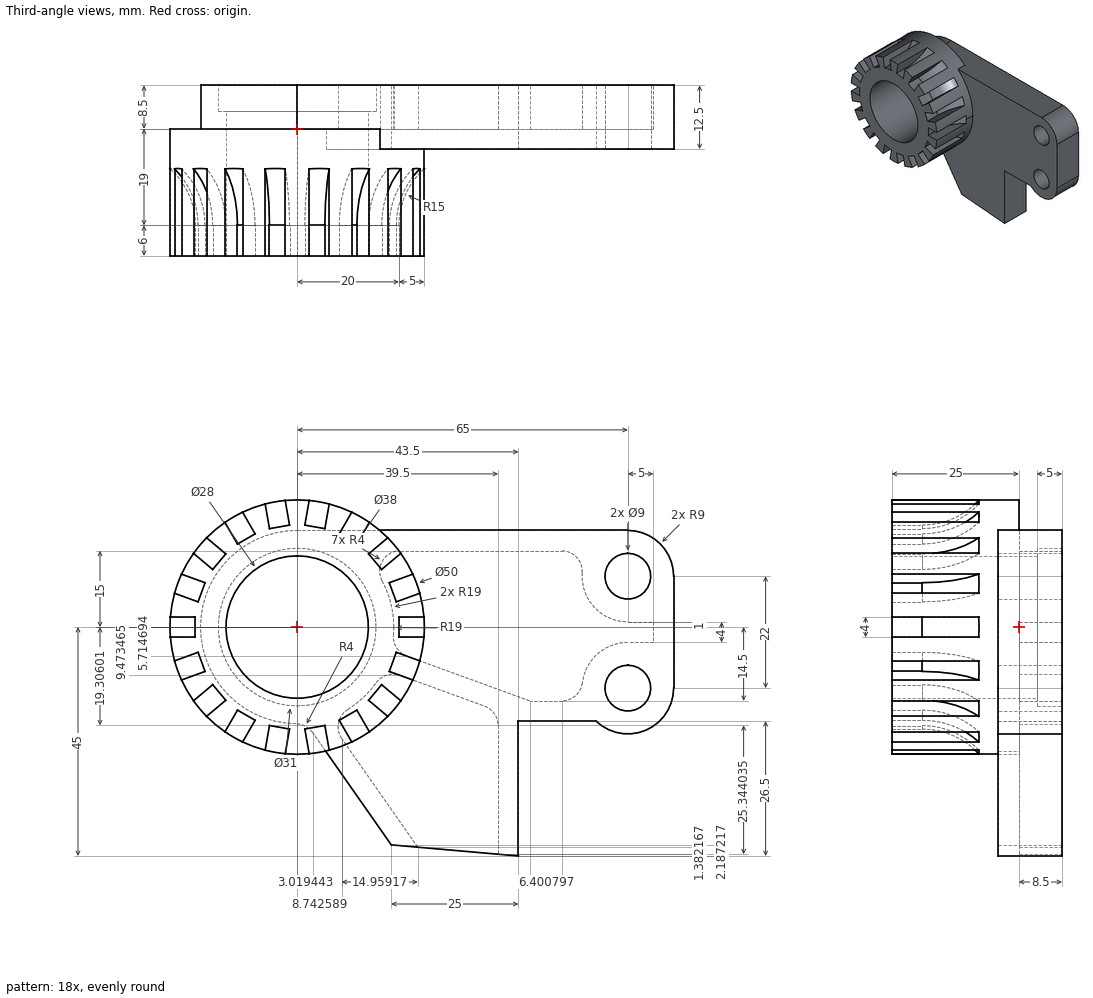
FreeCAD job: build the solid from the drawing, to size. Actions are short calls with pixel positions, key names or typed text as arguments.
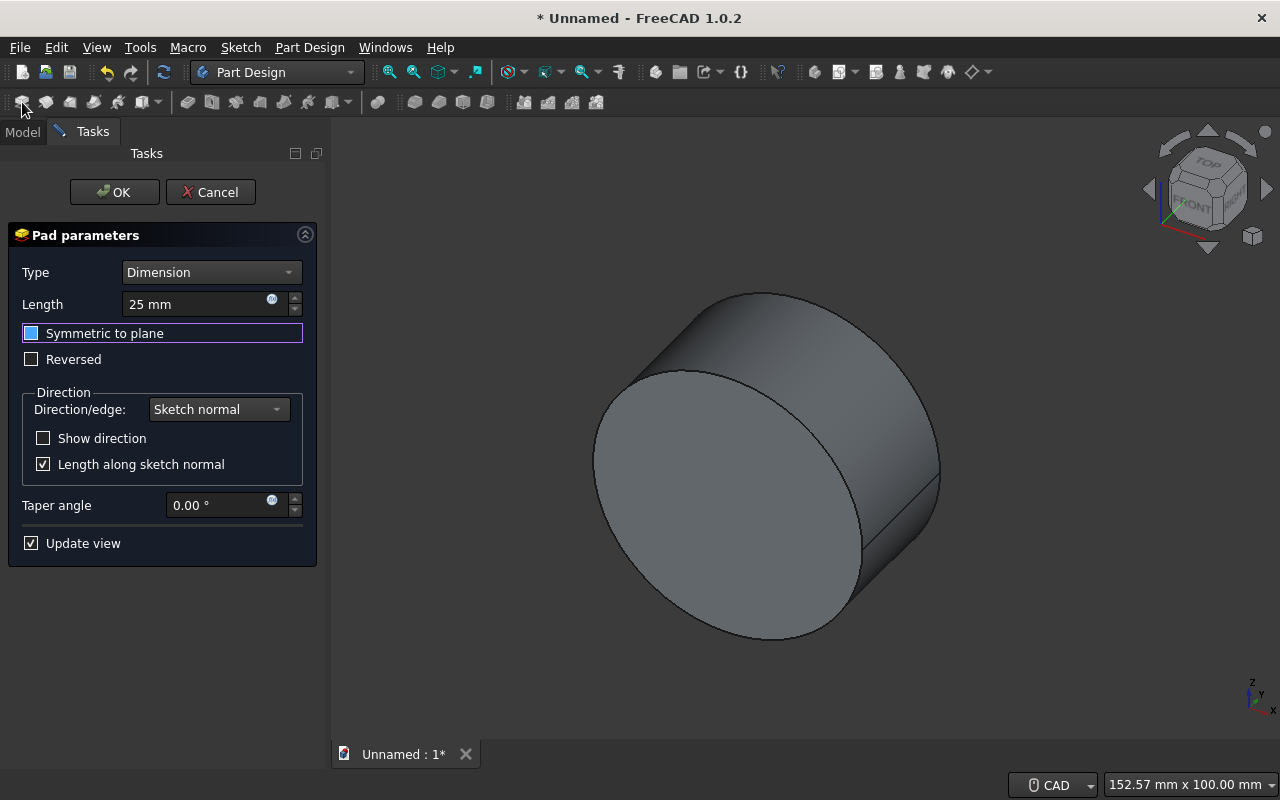
click(115, 192)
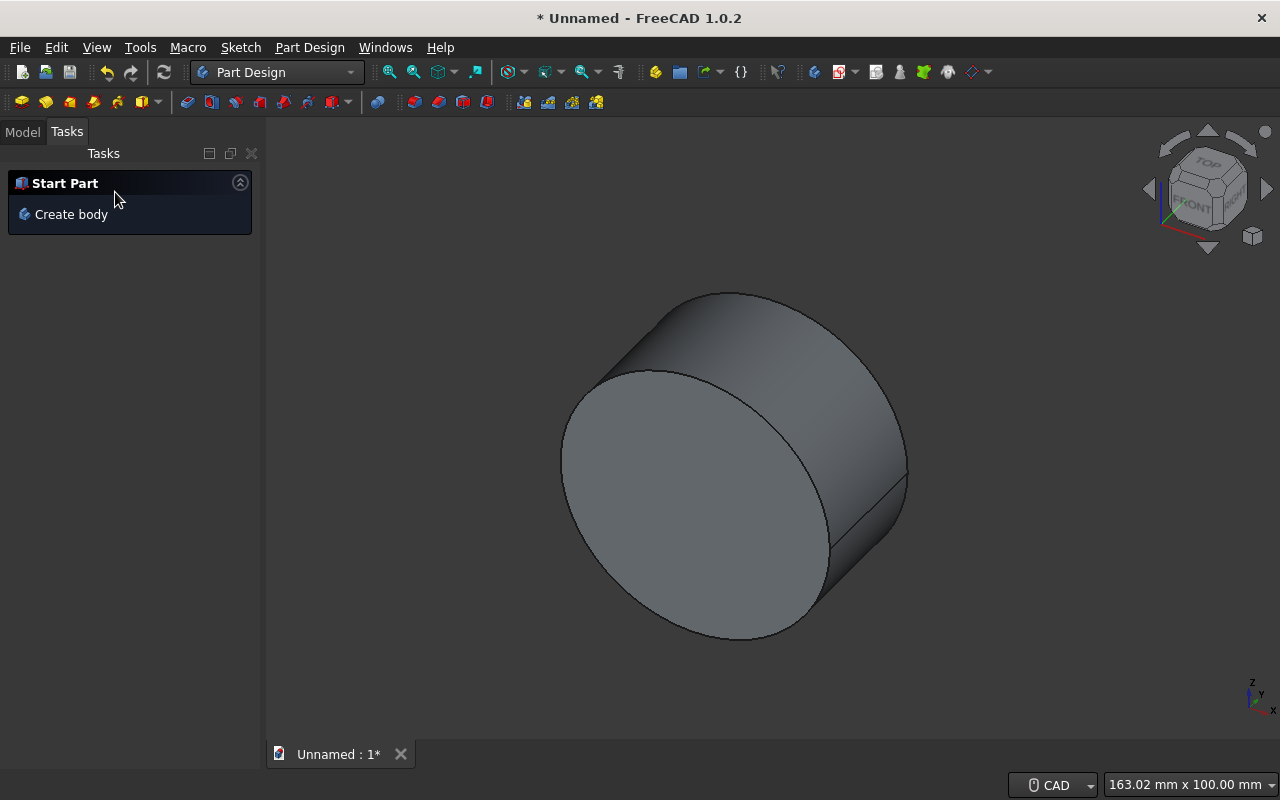
key(4)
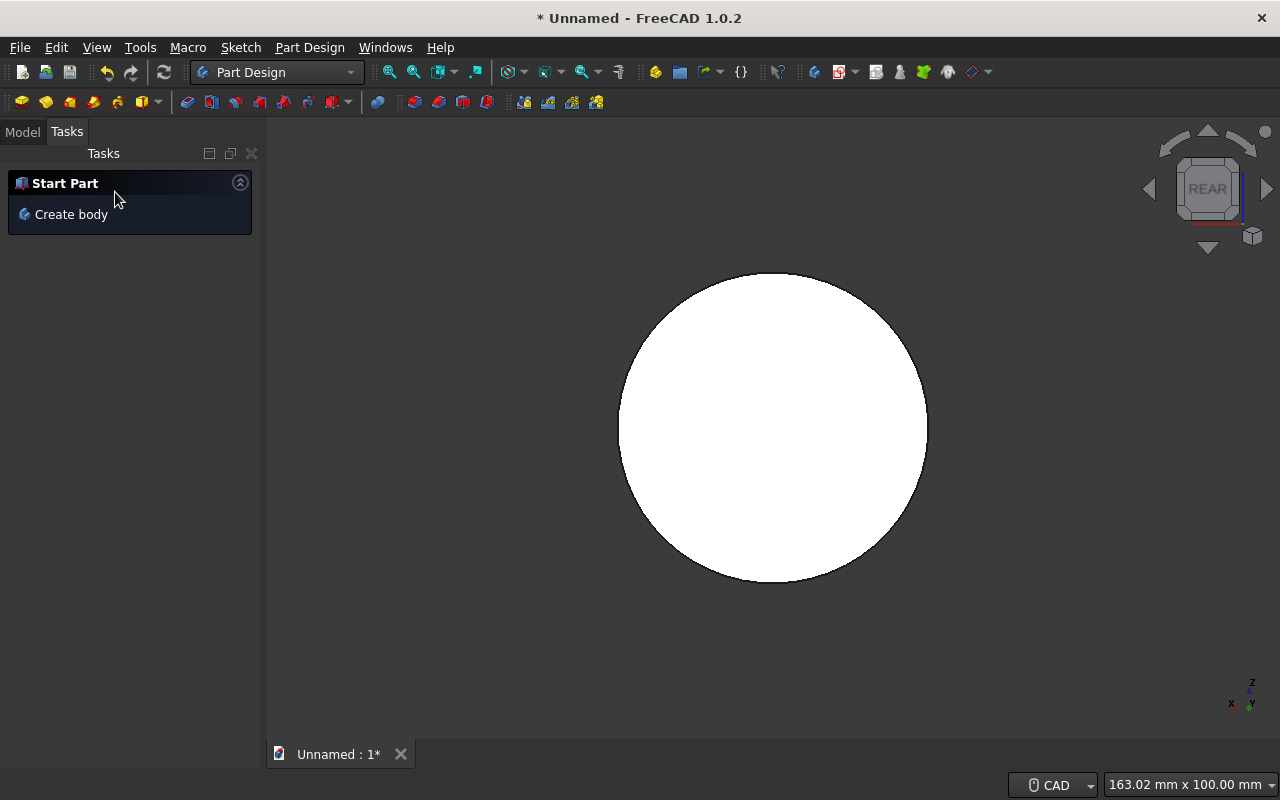
click(773, 427)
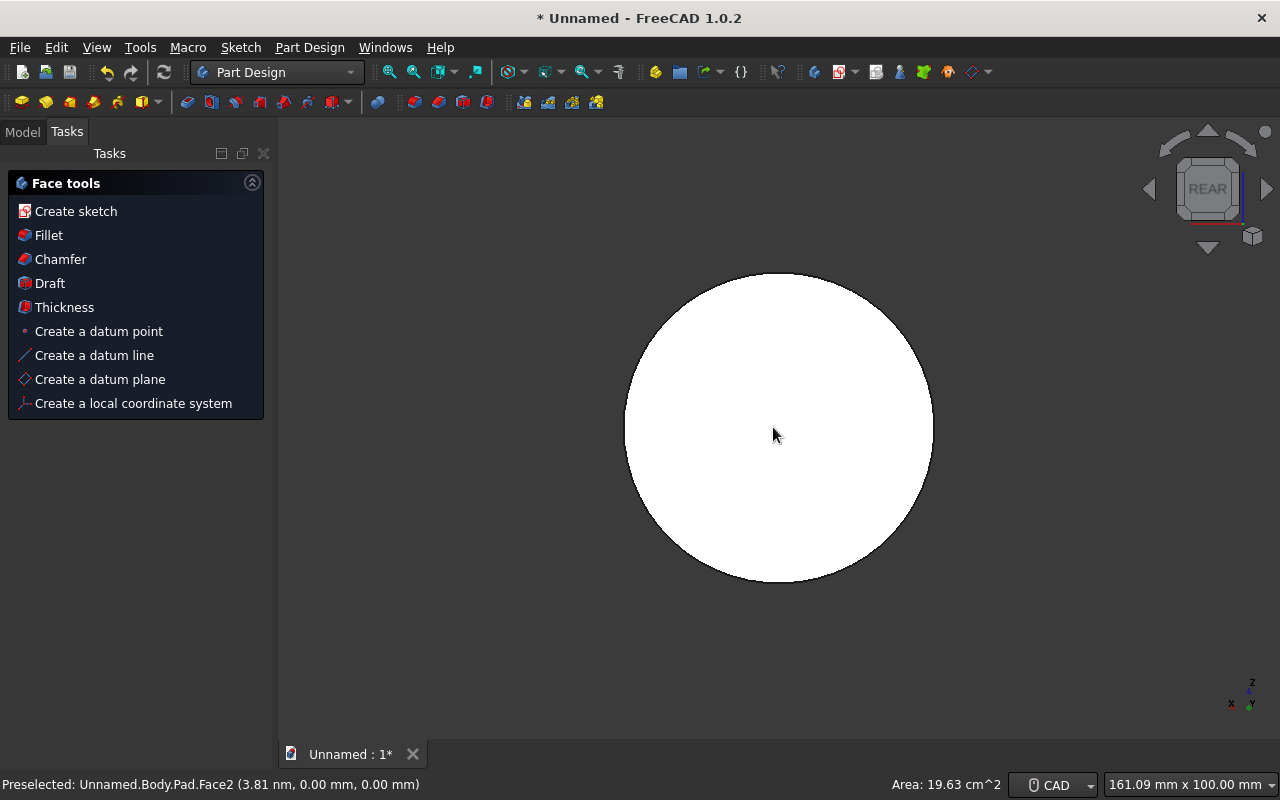
click(840, 72)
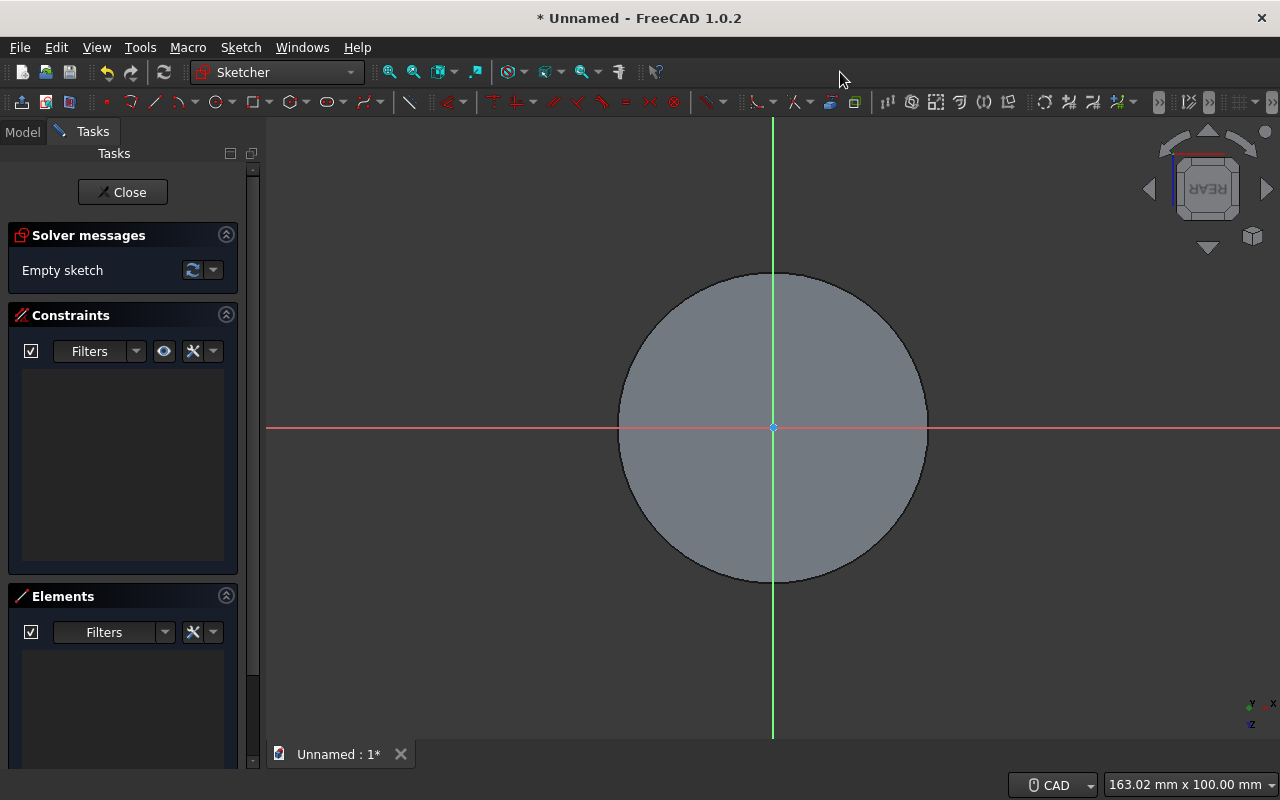
scroll(856, 428, up, 3)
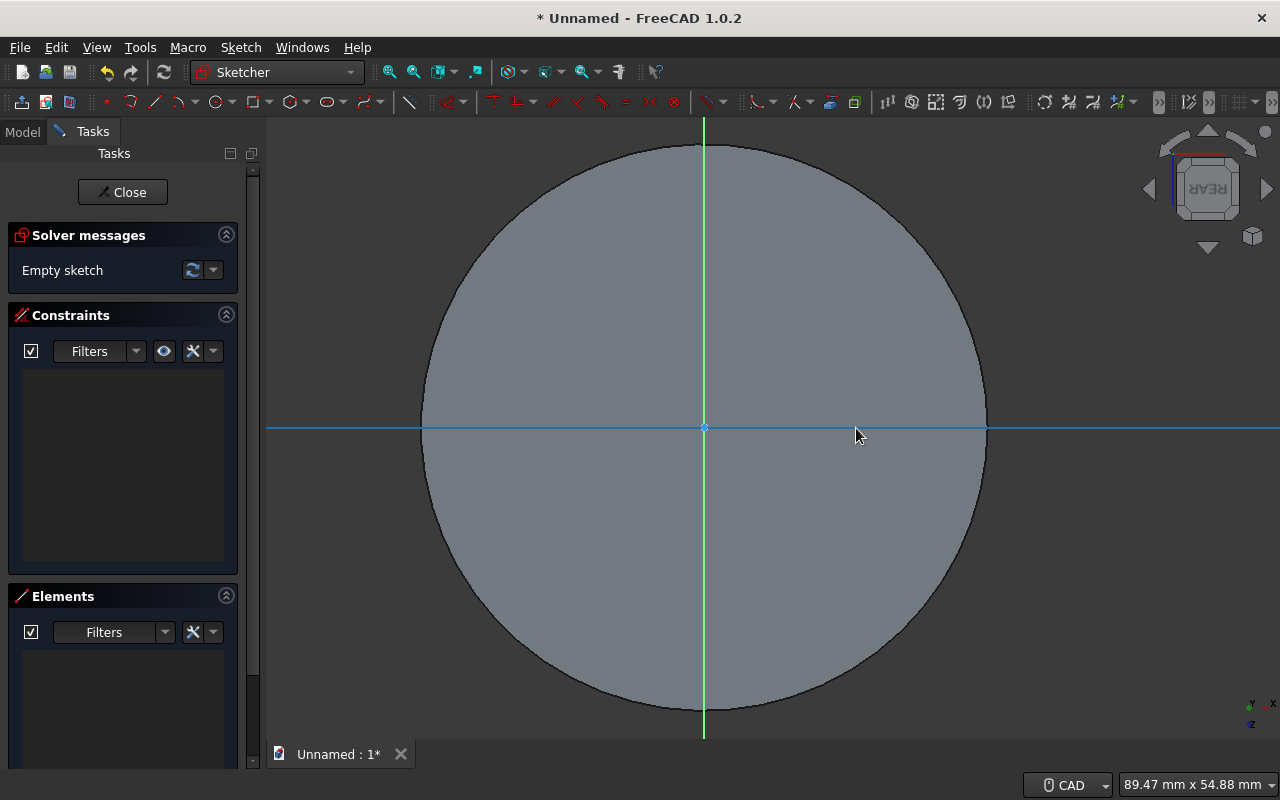
click(216, 102)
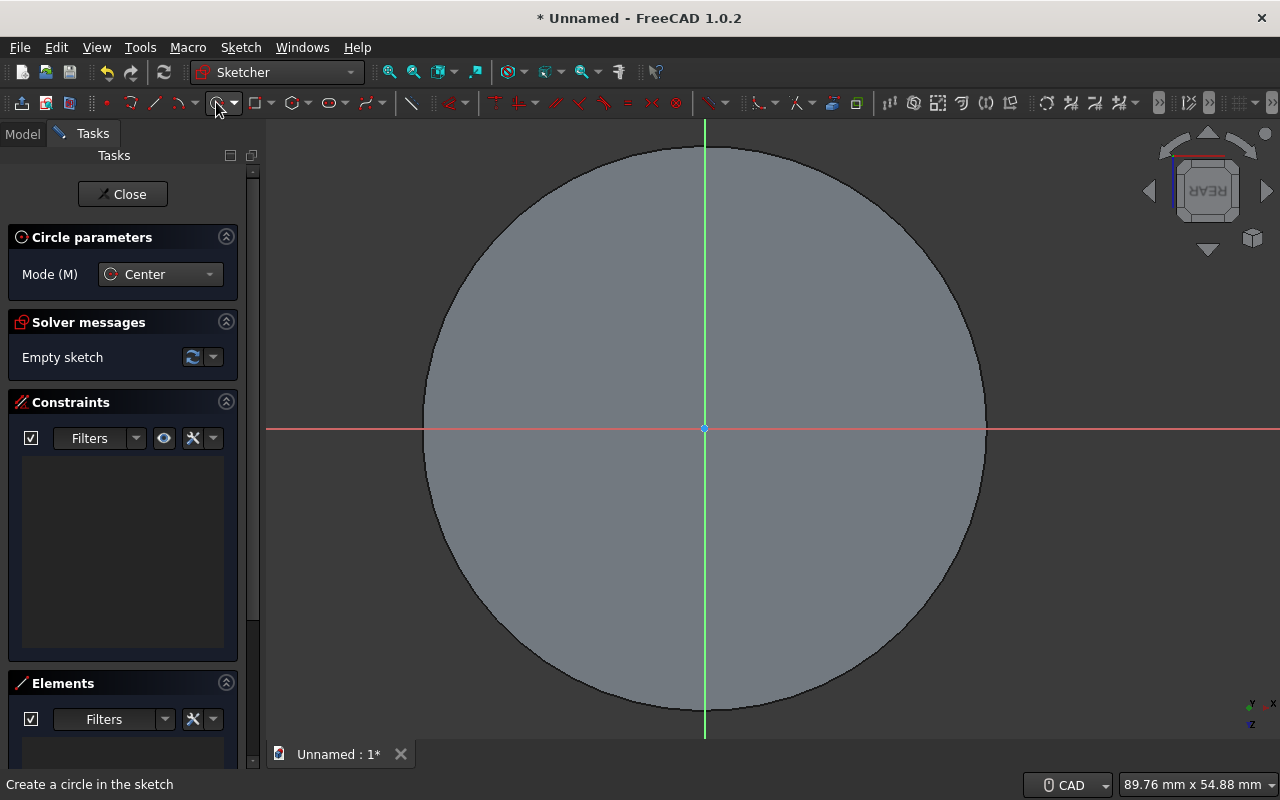
click(705, 429)
move(856, 277)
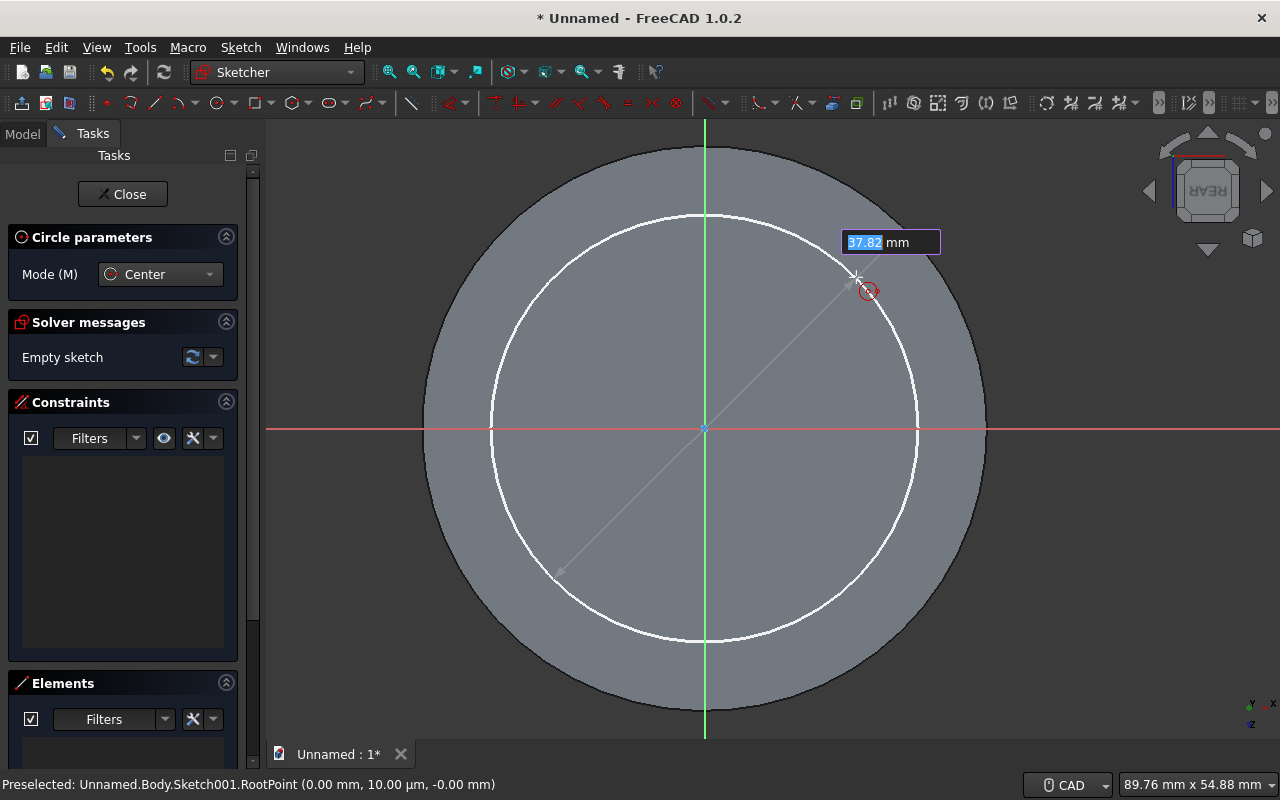
text(38)
key(Return)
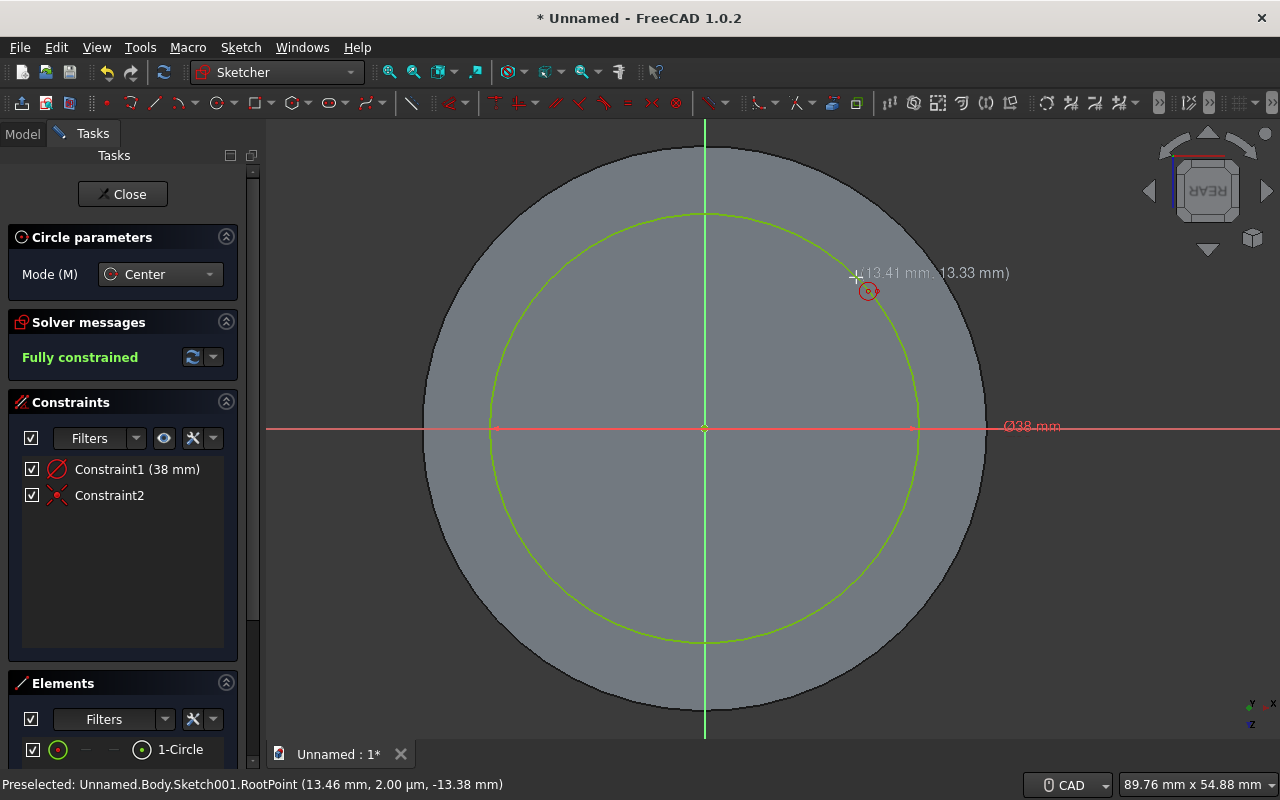
click(705, 429)
move(816, 317)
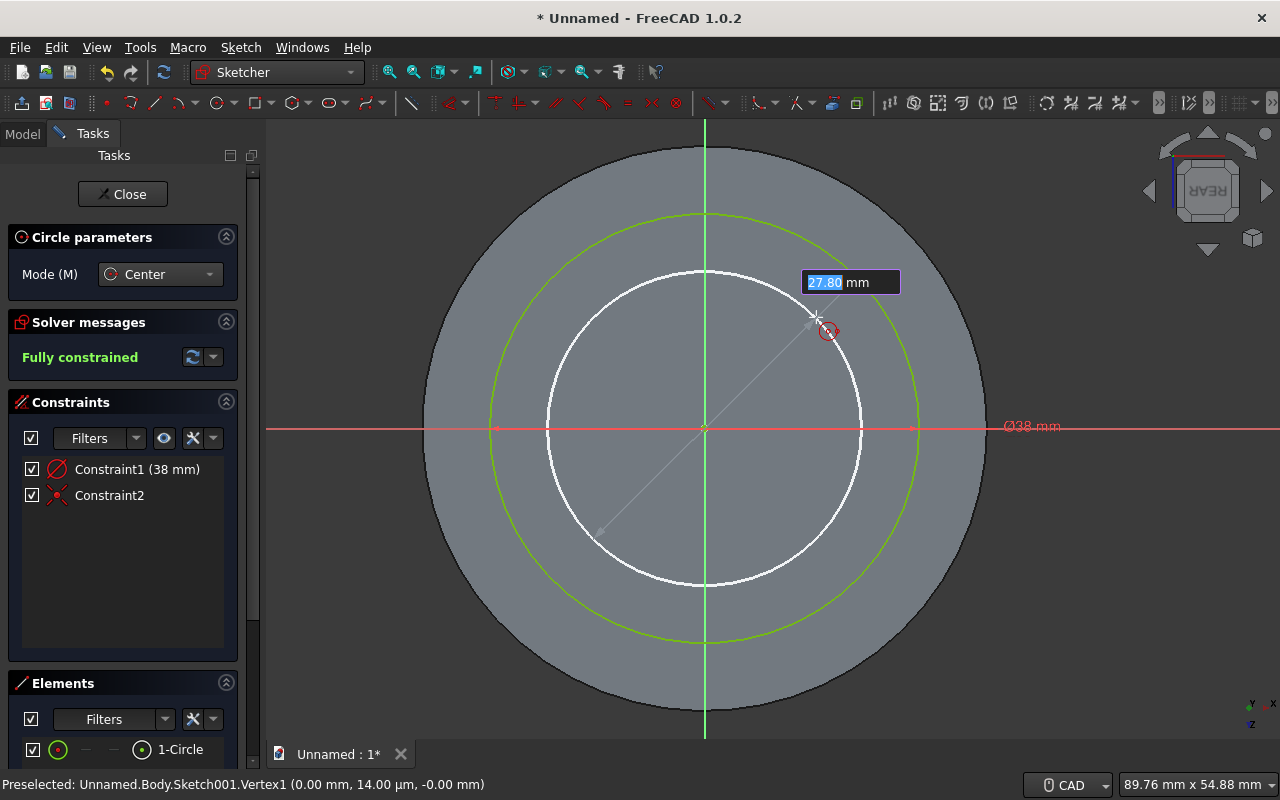
text(28)
key(Return)
key(Escape)